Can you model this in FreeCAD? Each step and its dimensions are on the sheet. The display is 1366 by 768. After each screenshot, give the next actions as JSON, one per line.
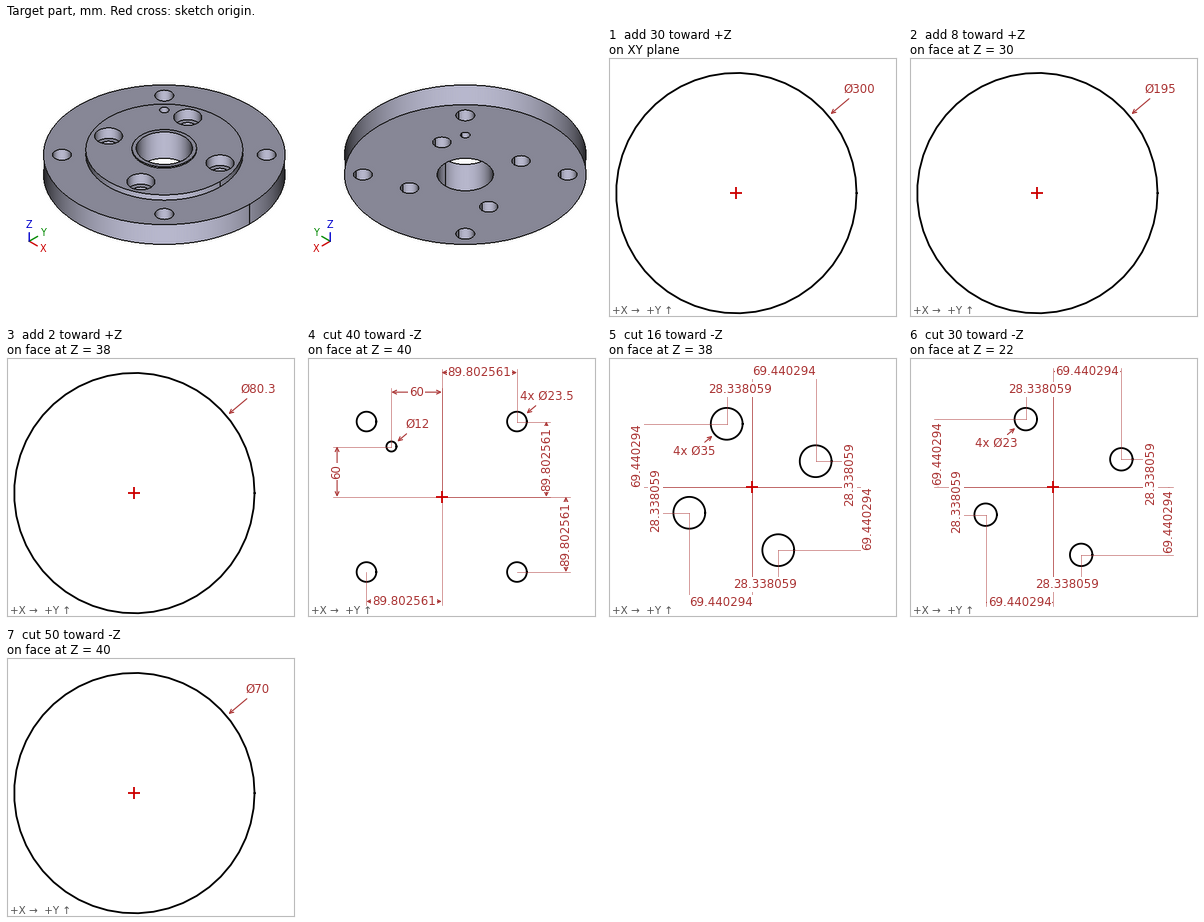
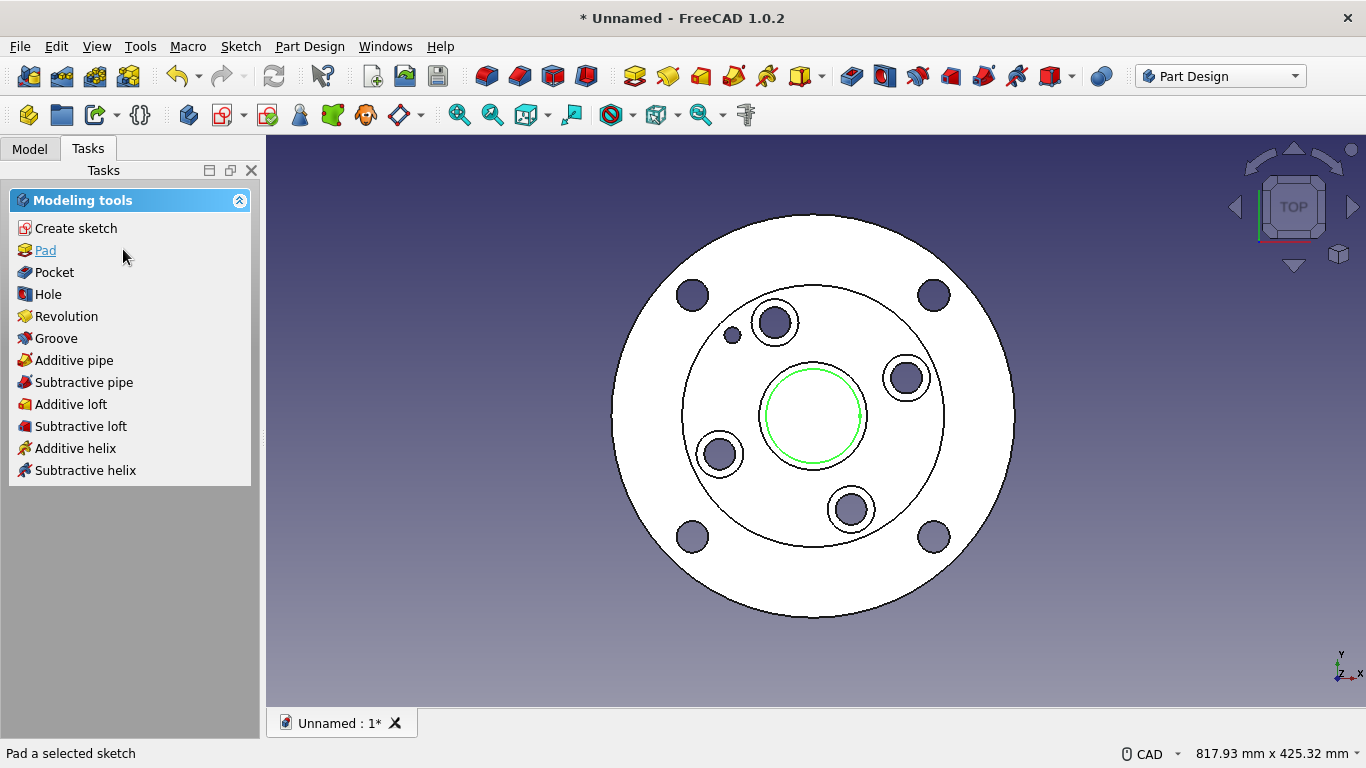
{"action": "left_click", "coordinate": [852, 76]}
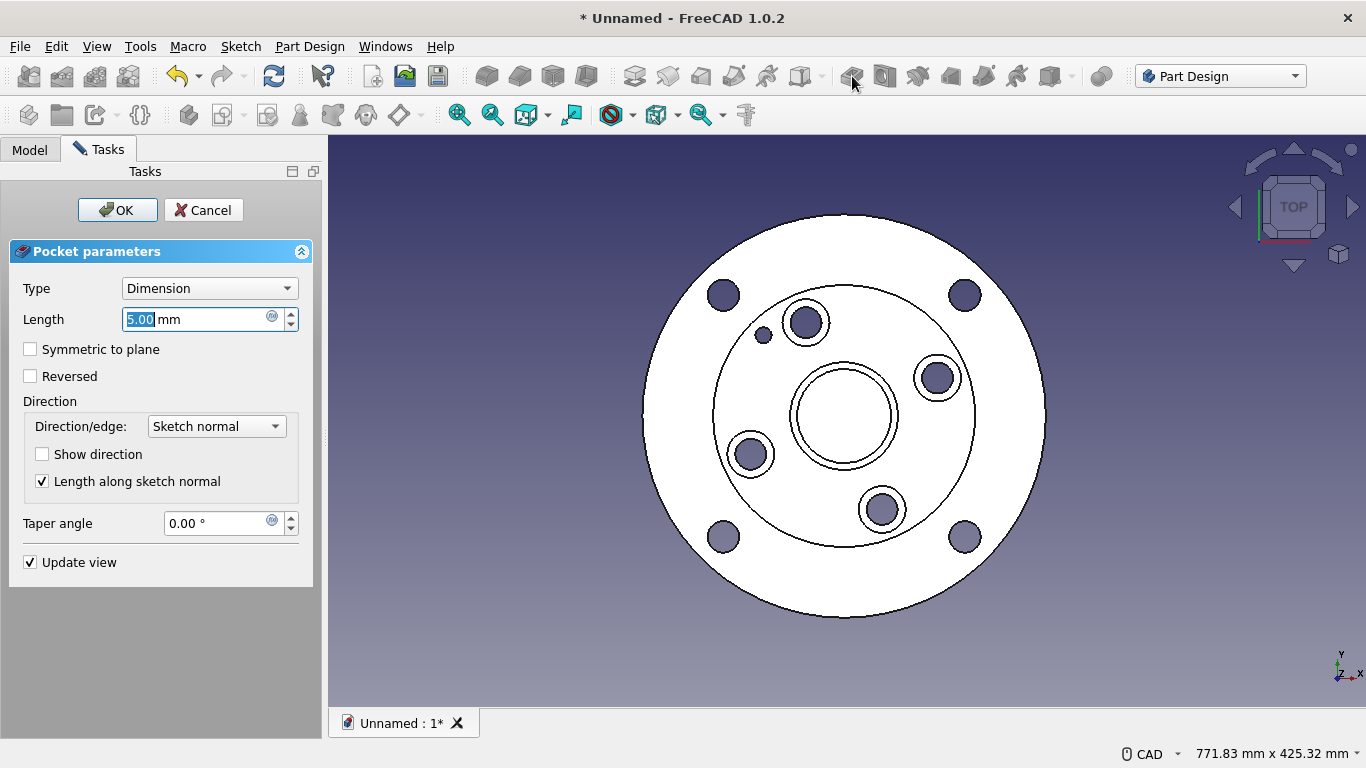
{"action": "type", "text": "50"}
{"action": "key", "text": "Tab"}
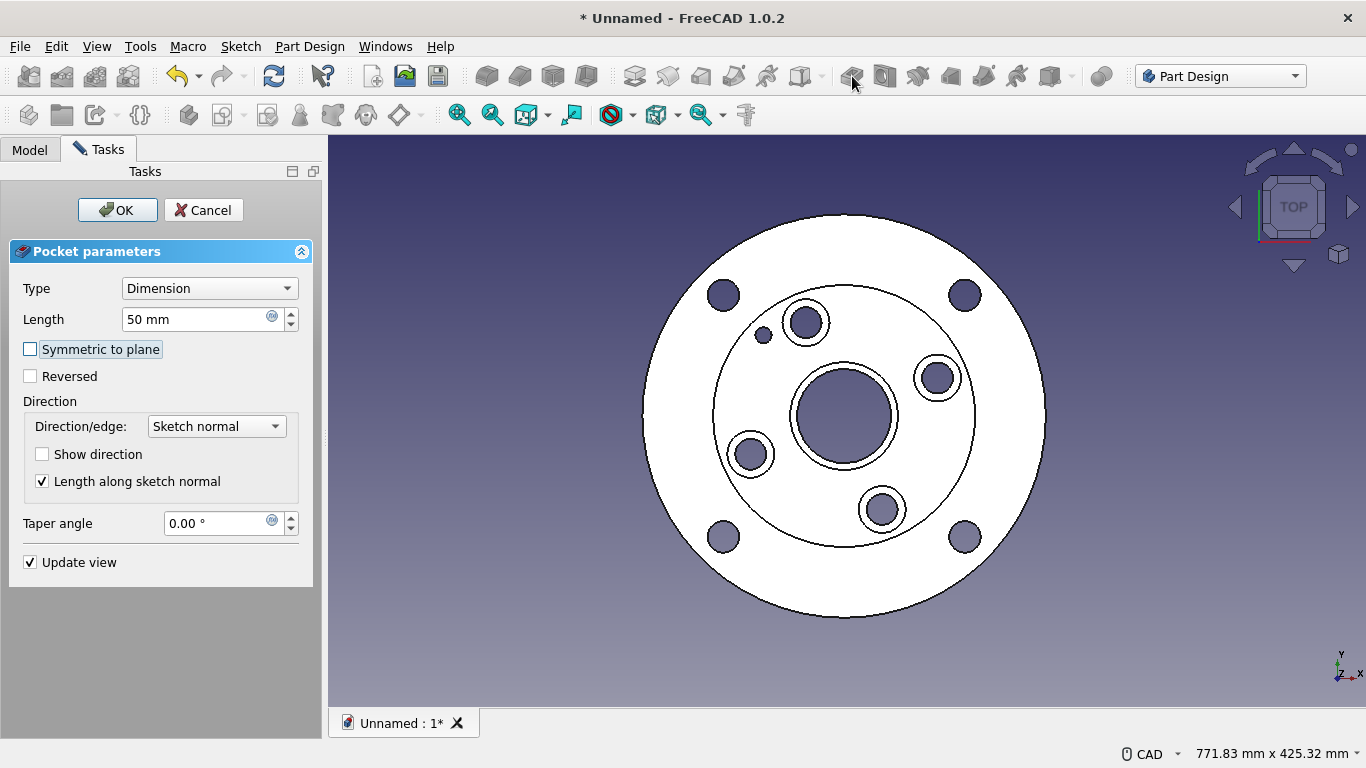
{"action": "left_click", "coordinate": [118, 210]}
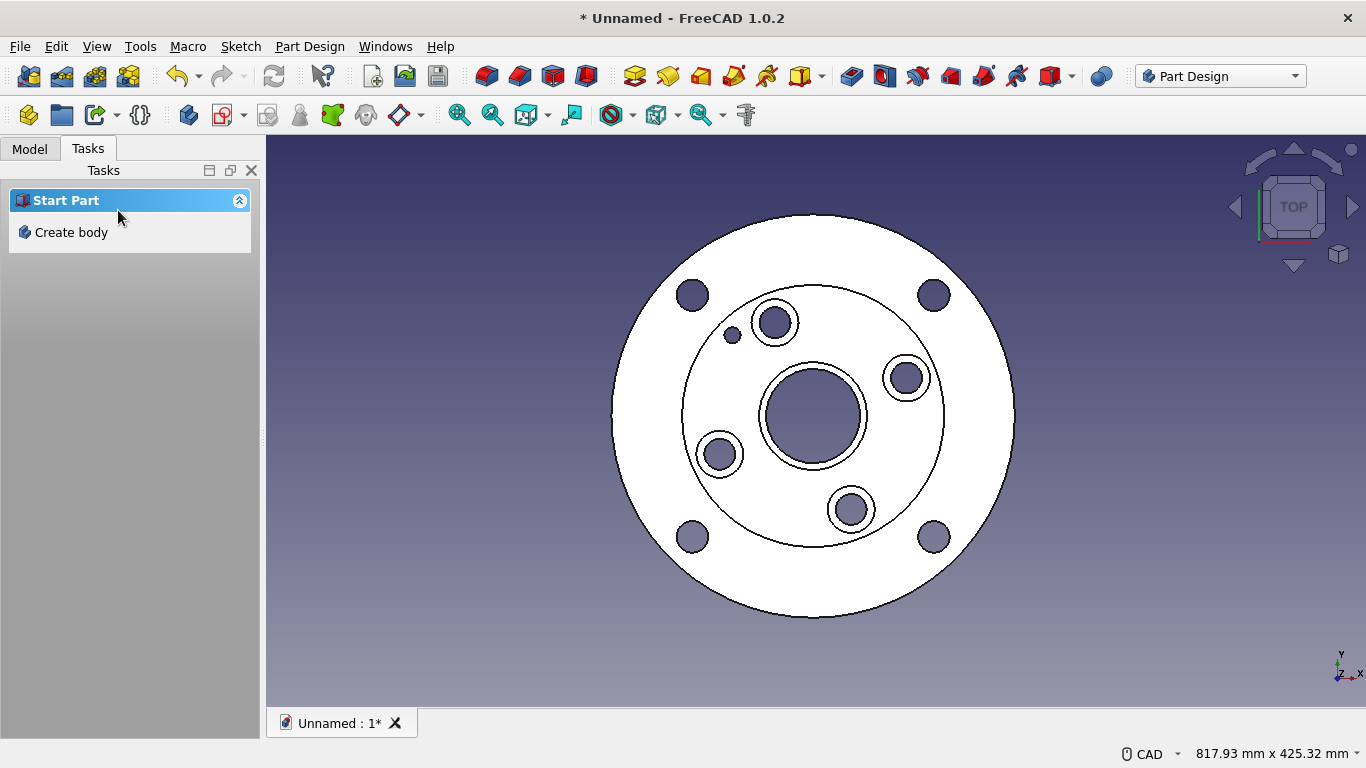
{"action": "key", "text": "0"}